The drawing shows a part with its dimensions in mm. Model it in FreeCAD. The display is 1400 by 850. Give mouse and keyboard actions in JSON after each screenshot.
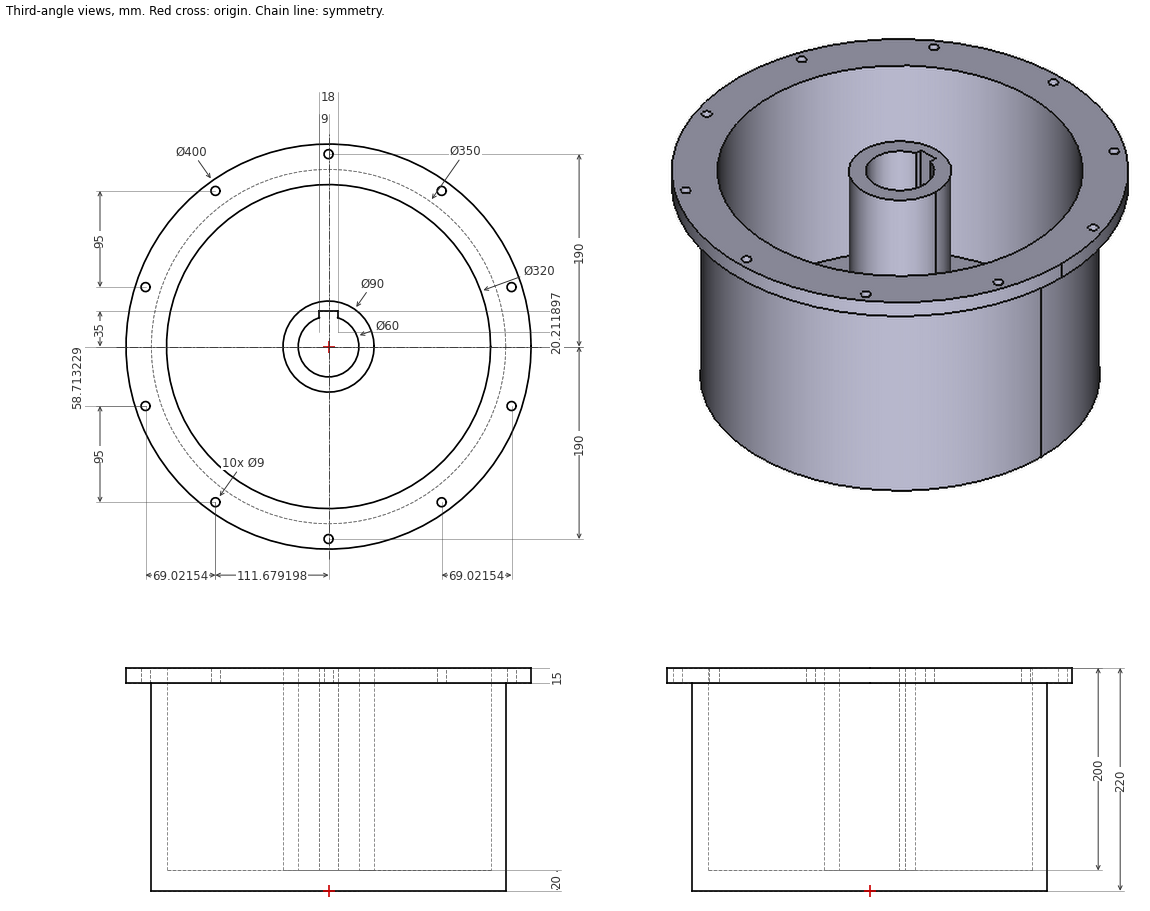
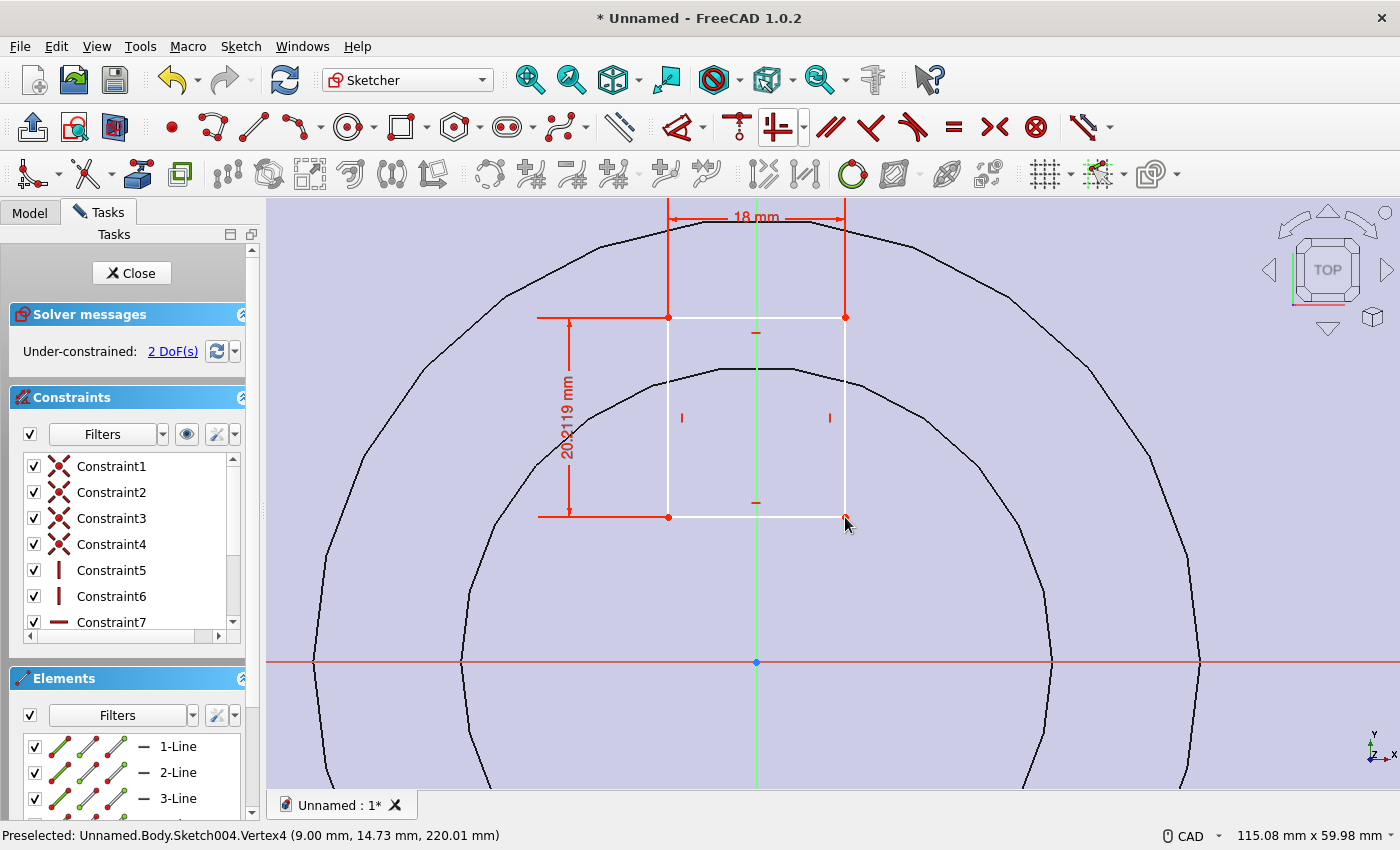
{"action": "left_click", "coordinate": [676, 128]}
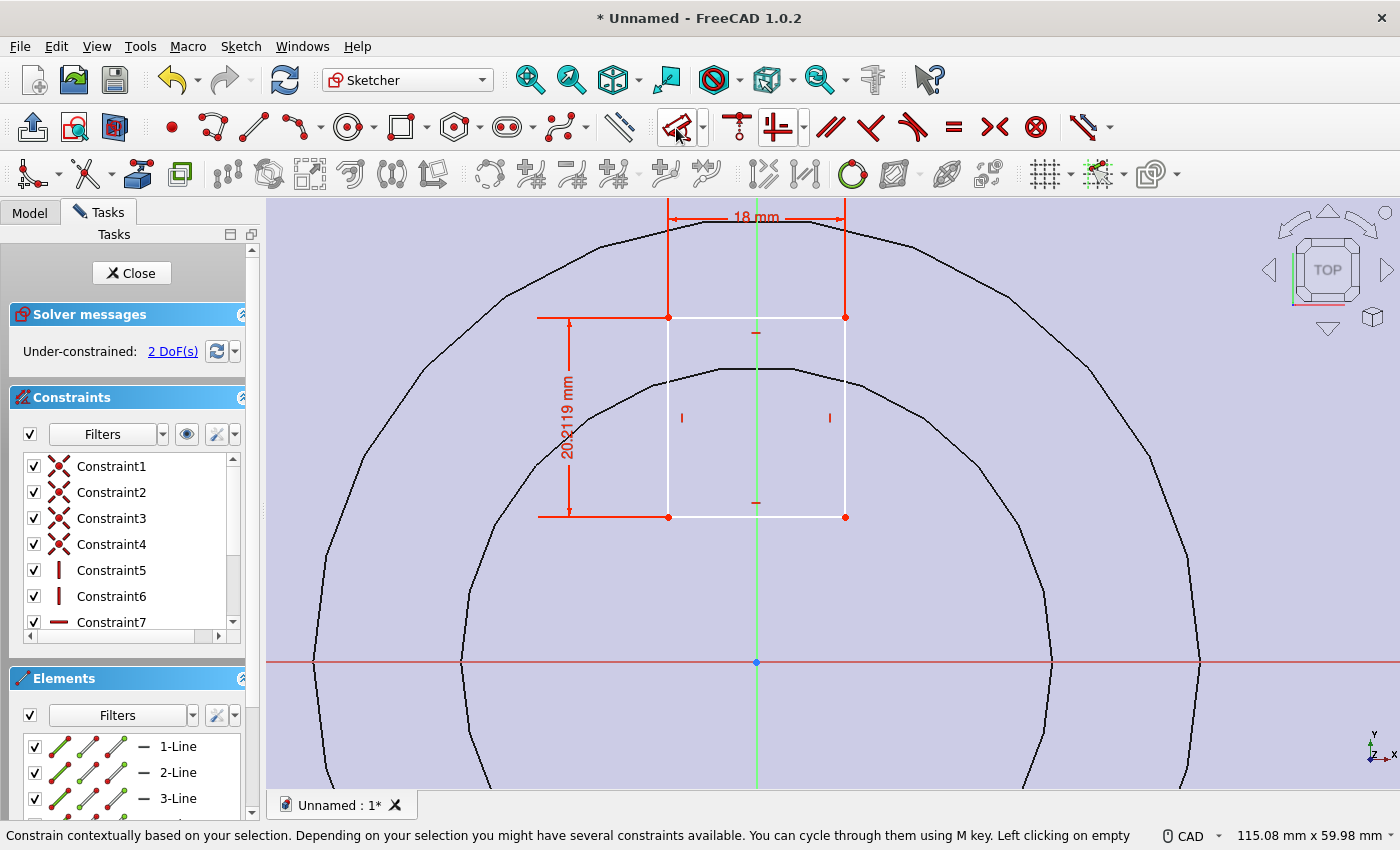
{"action": "left_click", "coordinate": [668, 318]}
{"action": "left_click", "coordinate": [712, 696]}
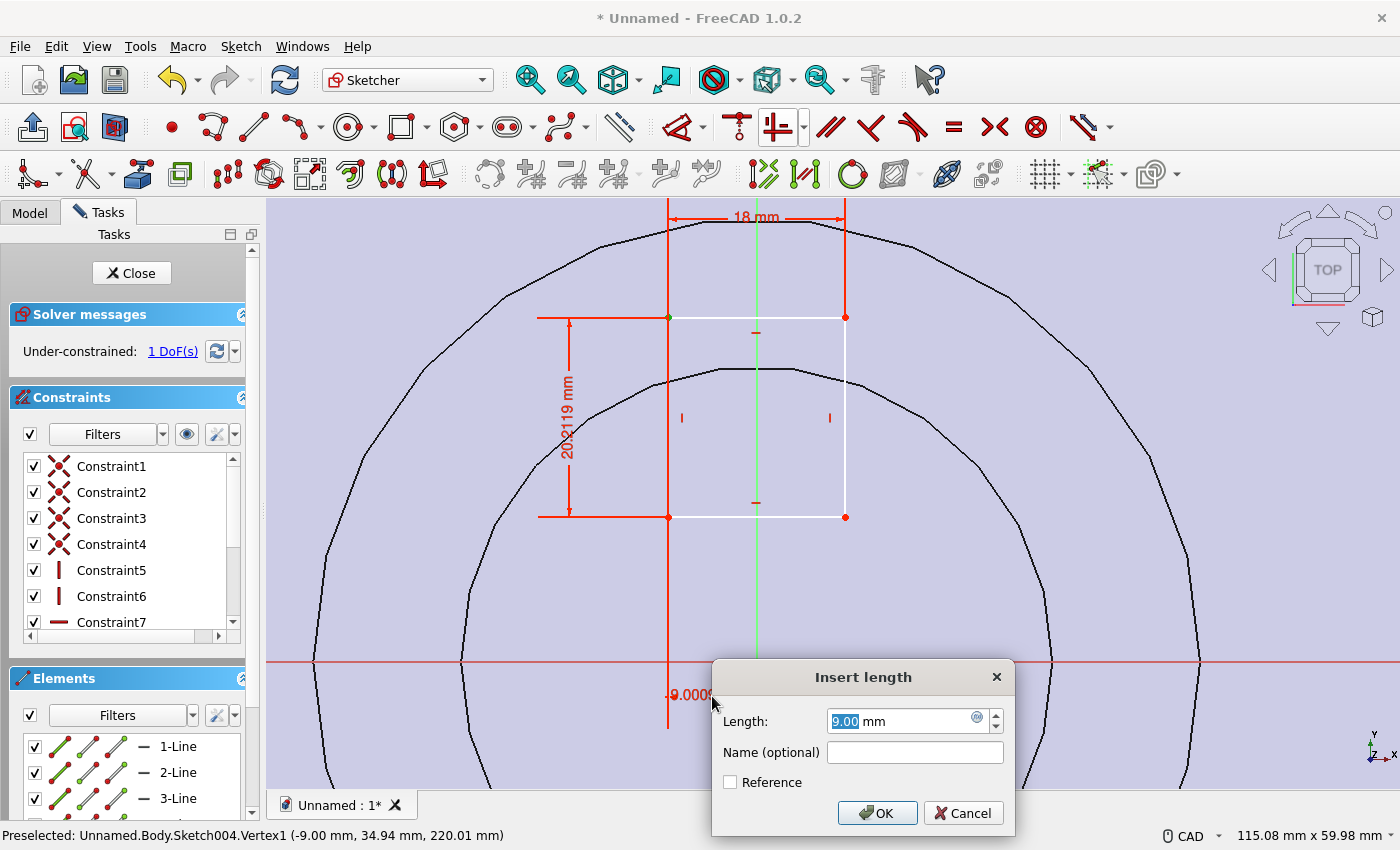
{"action": "type", "text": "9"}
{"action": "key", "text": "Return"}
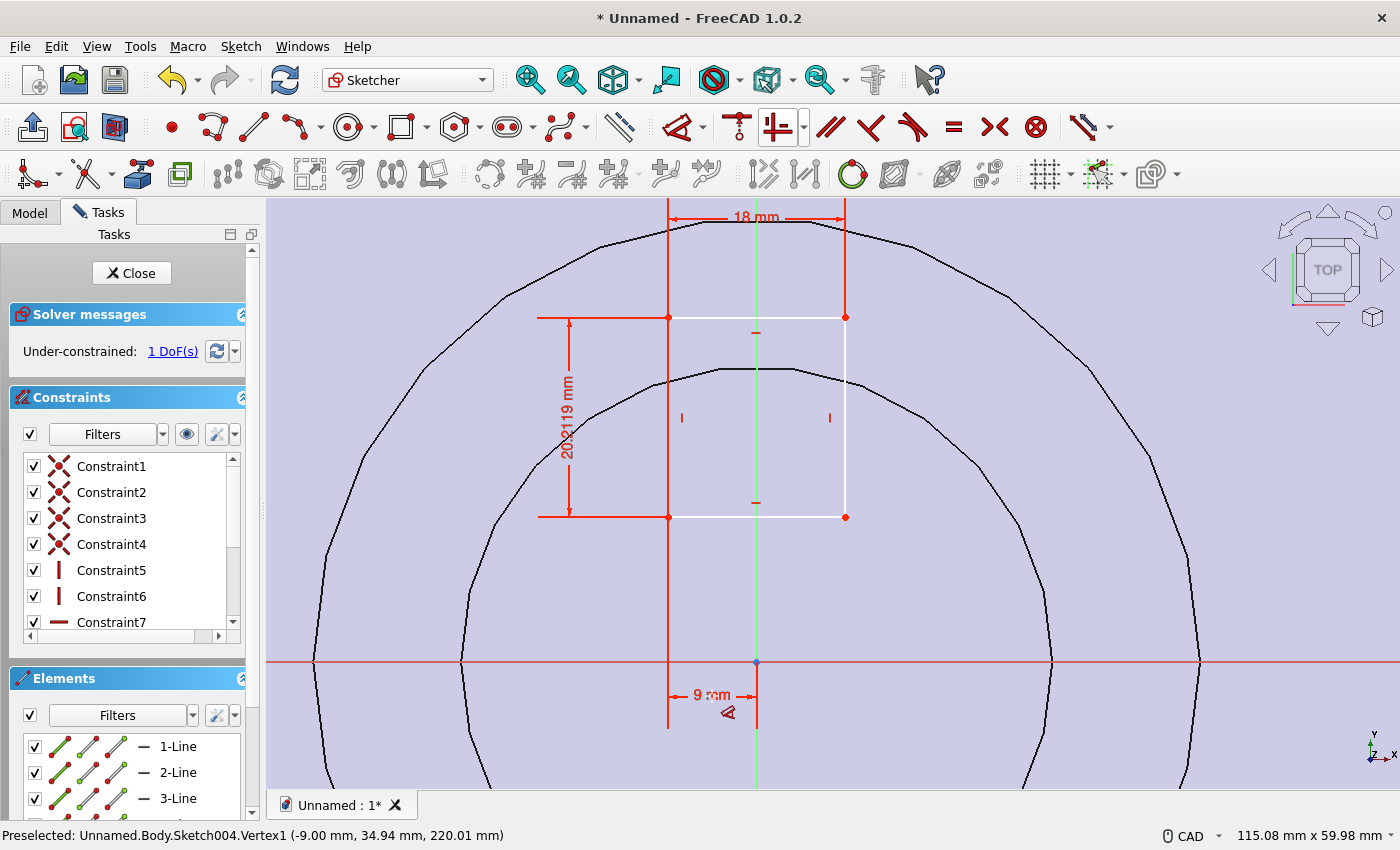
{"action": "left_click", "coordinate": [668, 318]}
{"action": "left_click", "coordinate": [634, 490]}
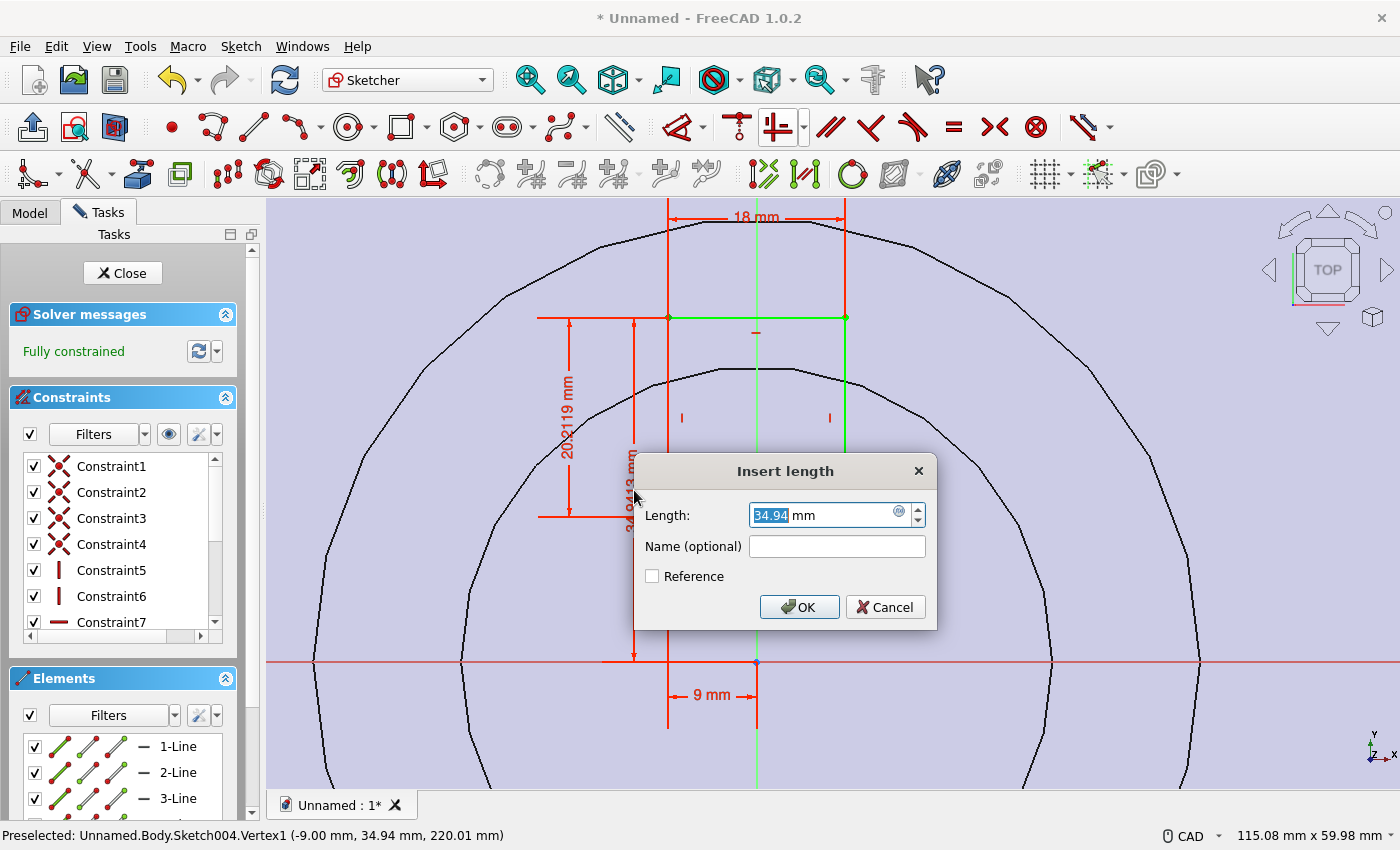
{"action": "type", "text": "35"}
{"action": "key", "text": "Return"}
{"action": "key", "text": "Escape"}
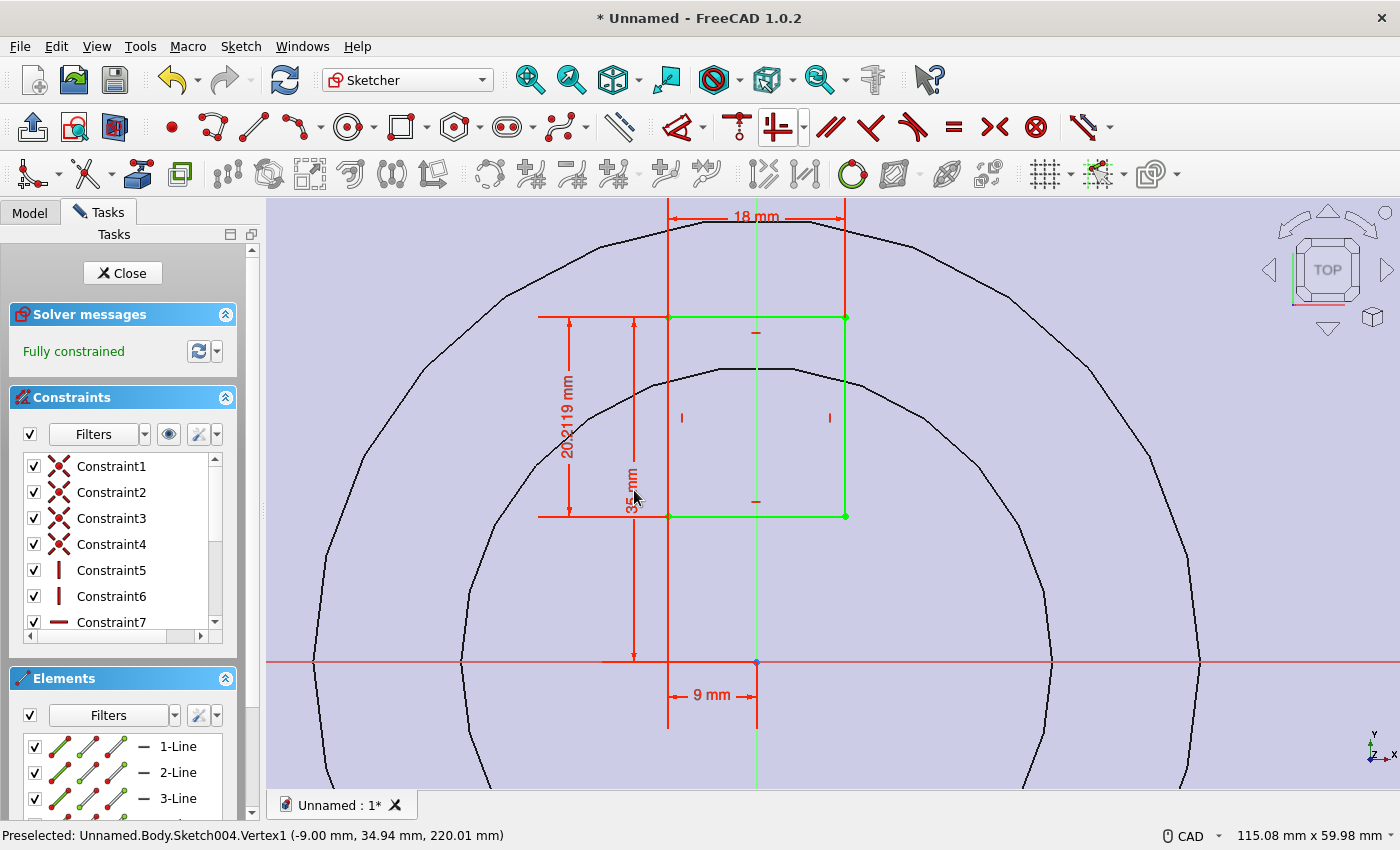
{"action": "left_click", "coordinate": [123, 273]}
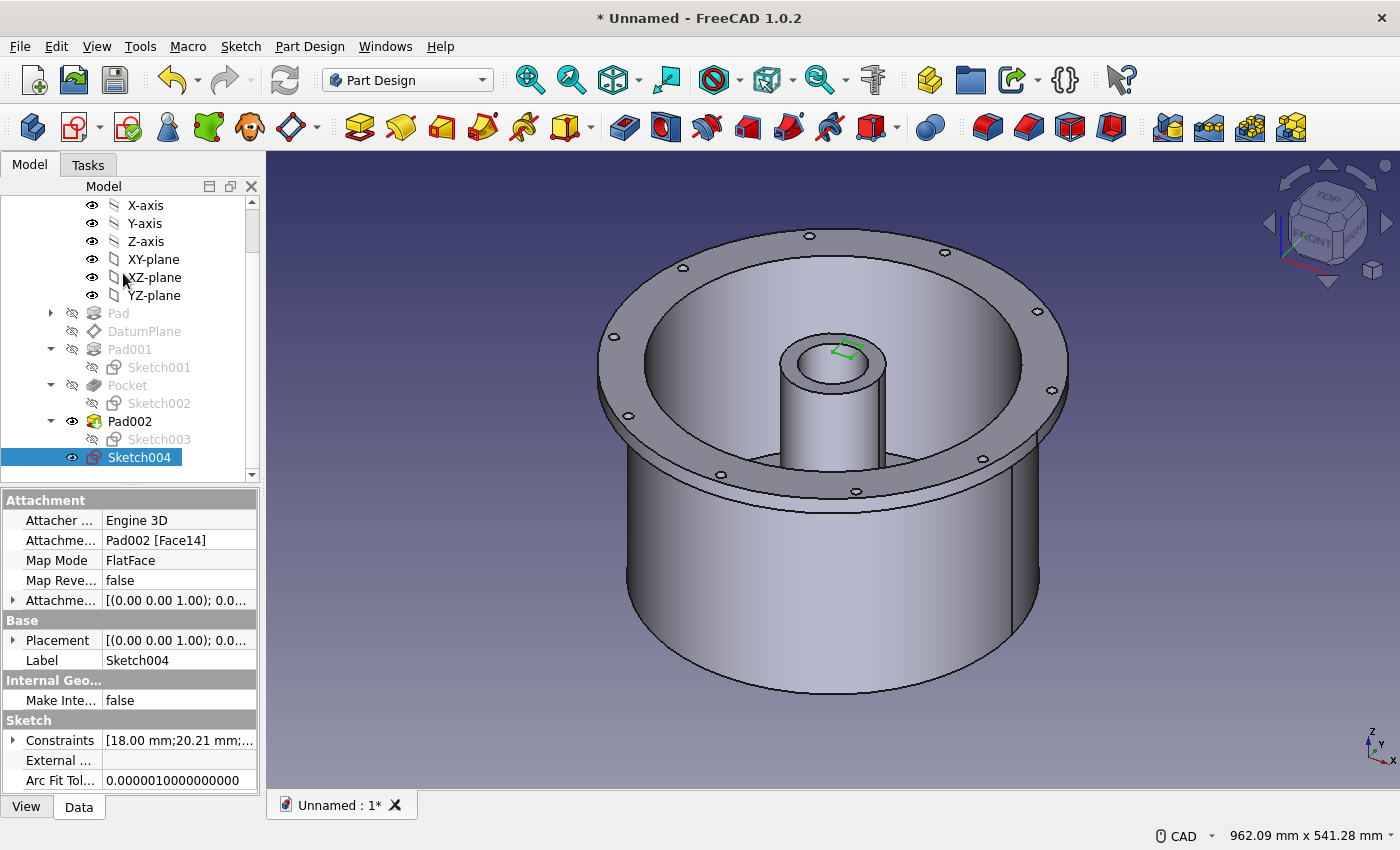
{"action": "left_click", "coordinate": [625, 128]}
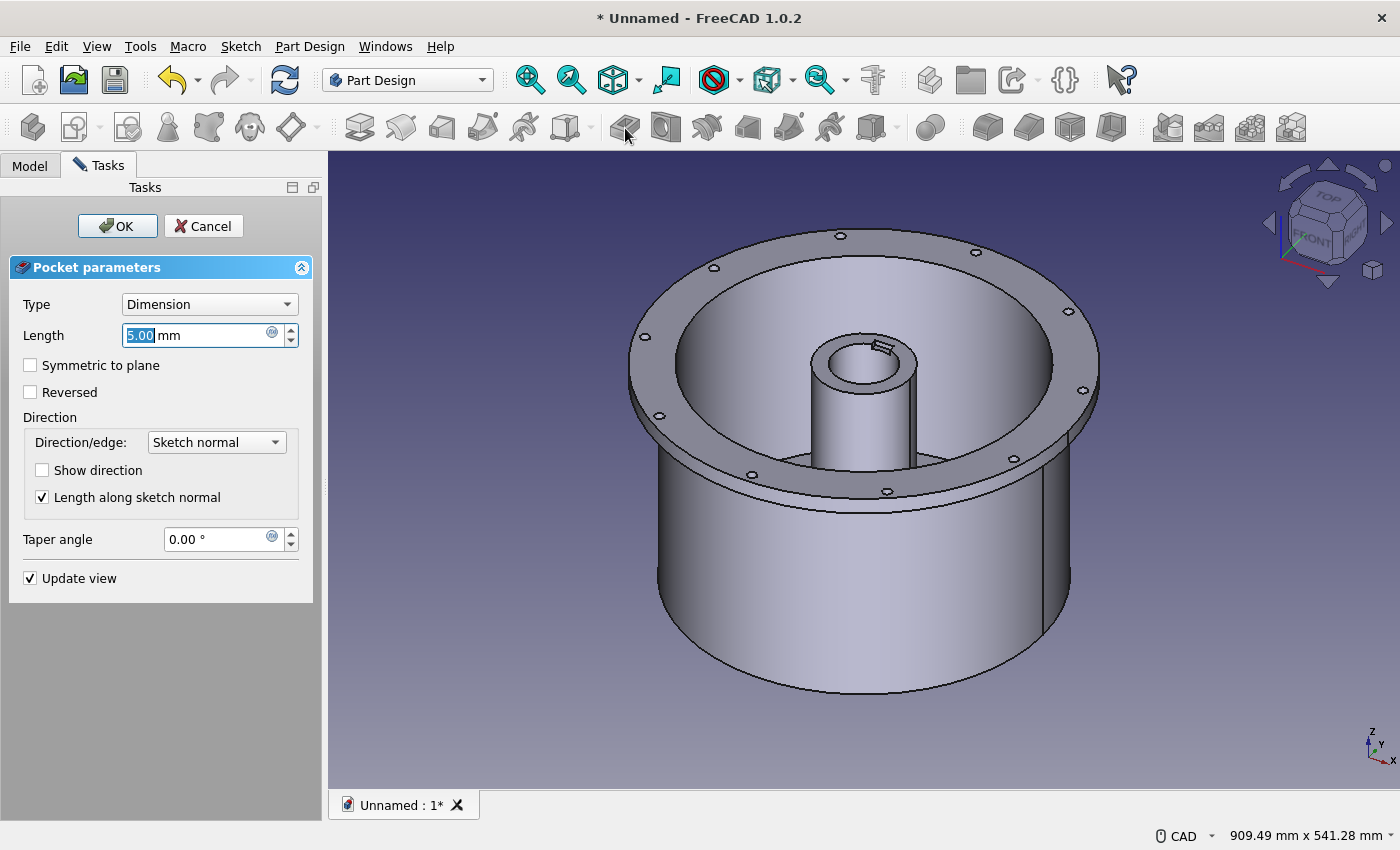
{"action": "type", "text": "200"}
{"action": "key", "text": "Tab"}